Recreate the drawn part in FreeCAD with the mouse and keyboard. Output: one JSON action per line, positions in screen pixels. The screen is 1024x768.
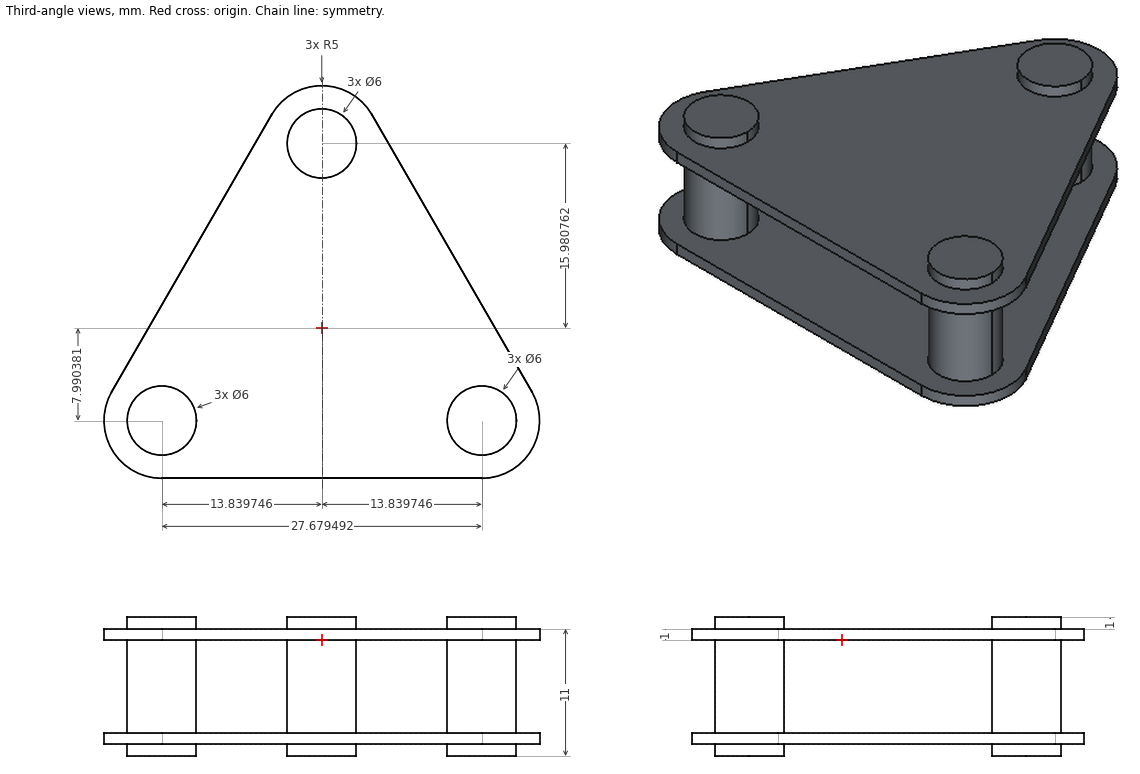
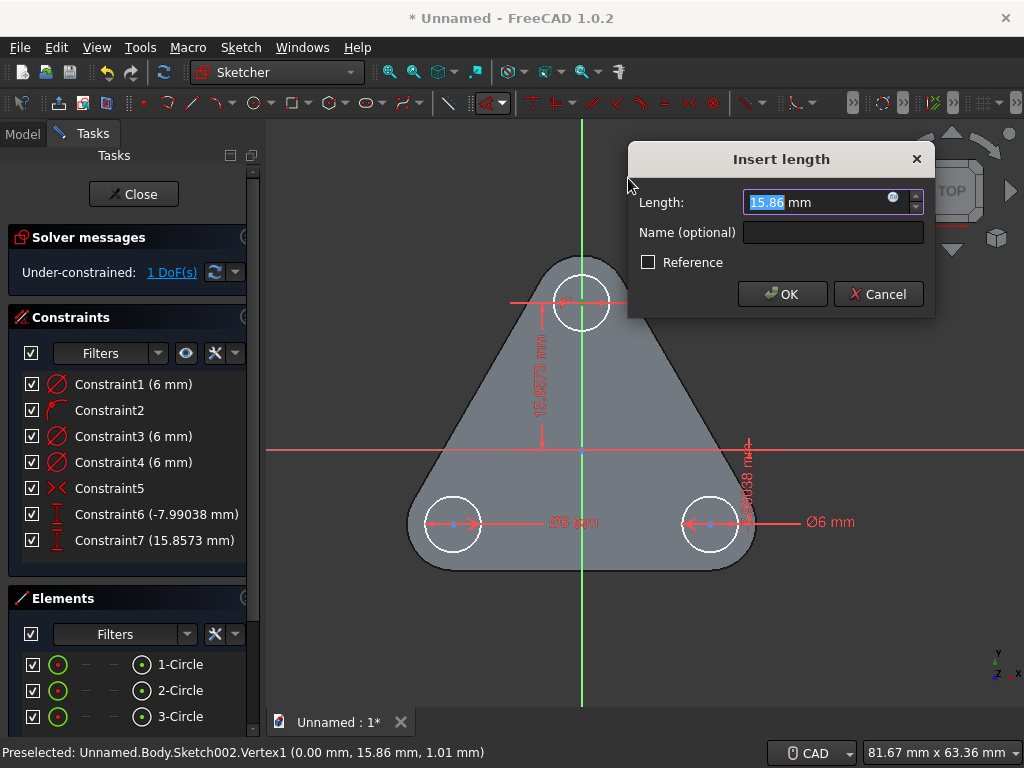
{"action": "type", "text": "15.980762"}
{"action": "key", "text": "Return"}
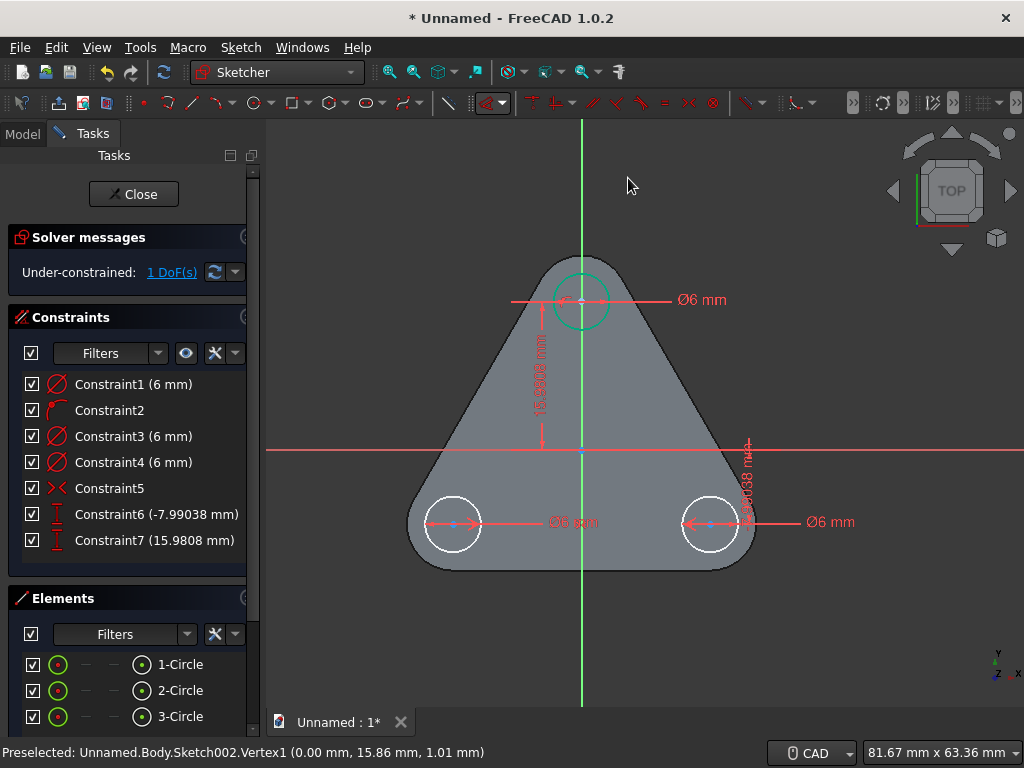
{"action": "left_click", "coordinate": [710, 524]}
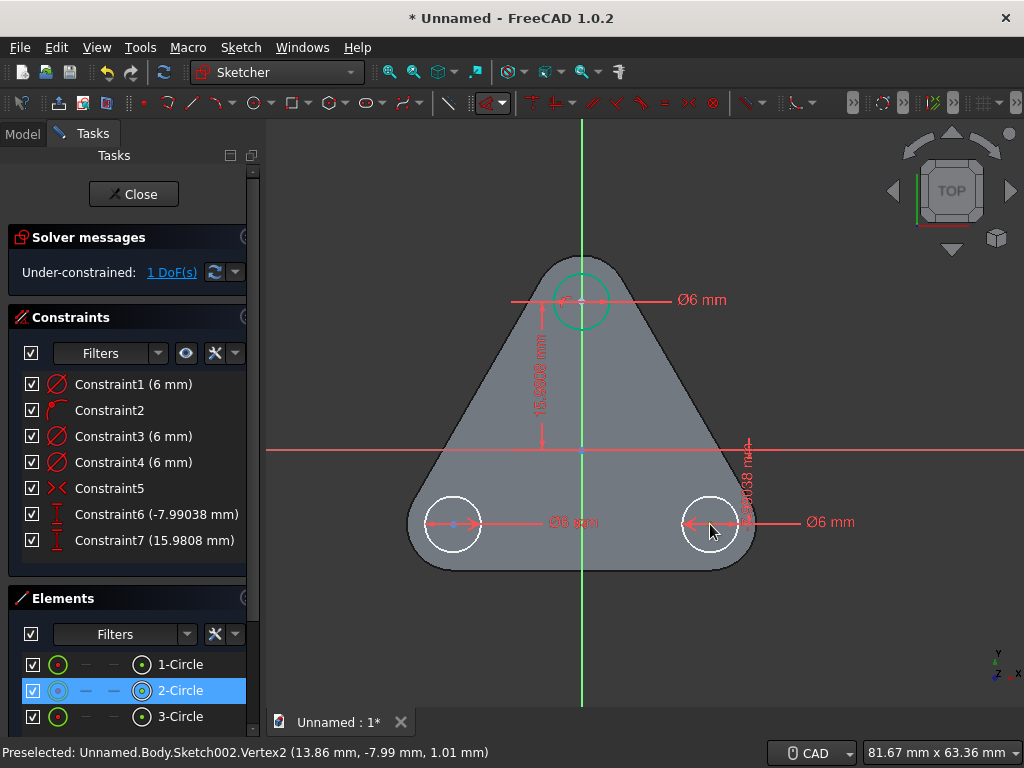
{"action": "left_click", "coordinate": [504, 104]}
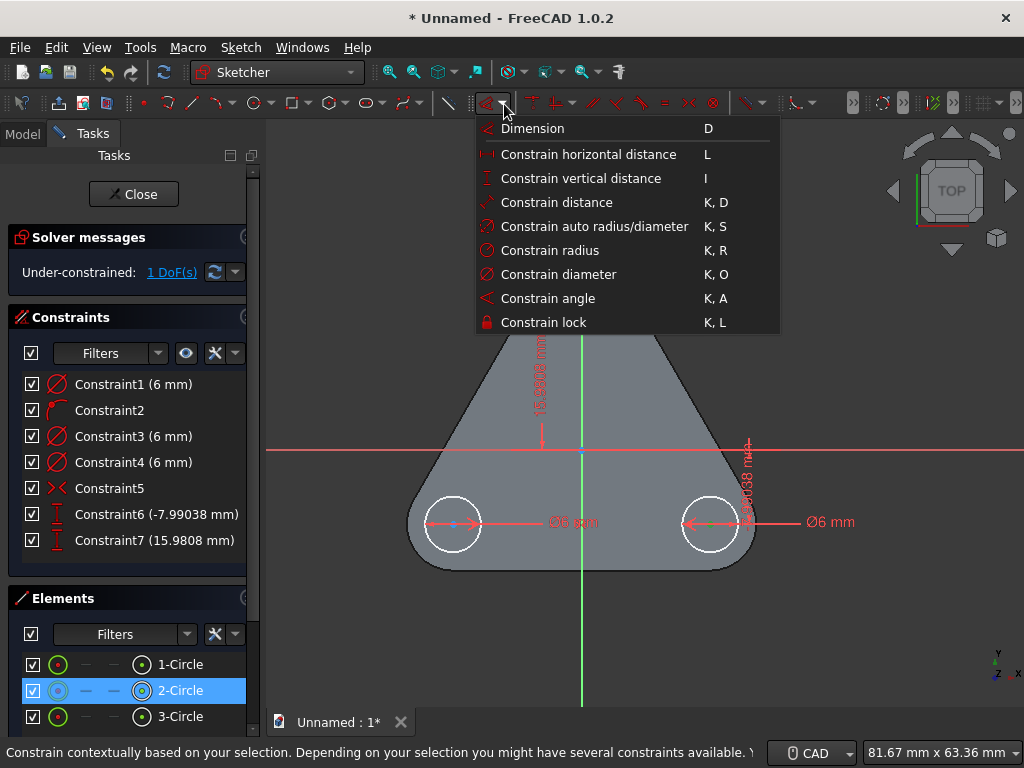
{"action": "left_click", "coordinate": [628, 154]}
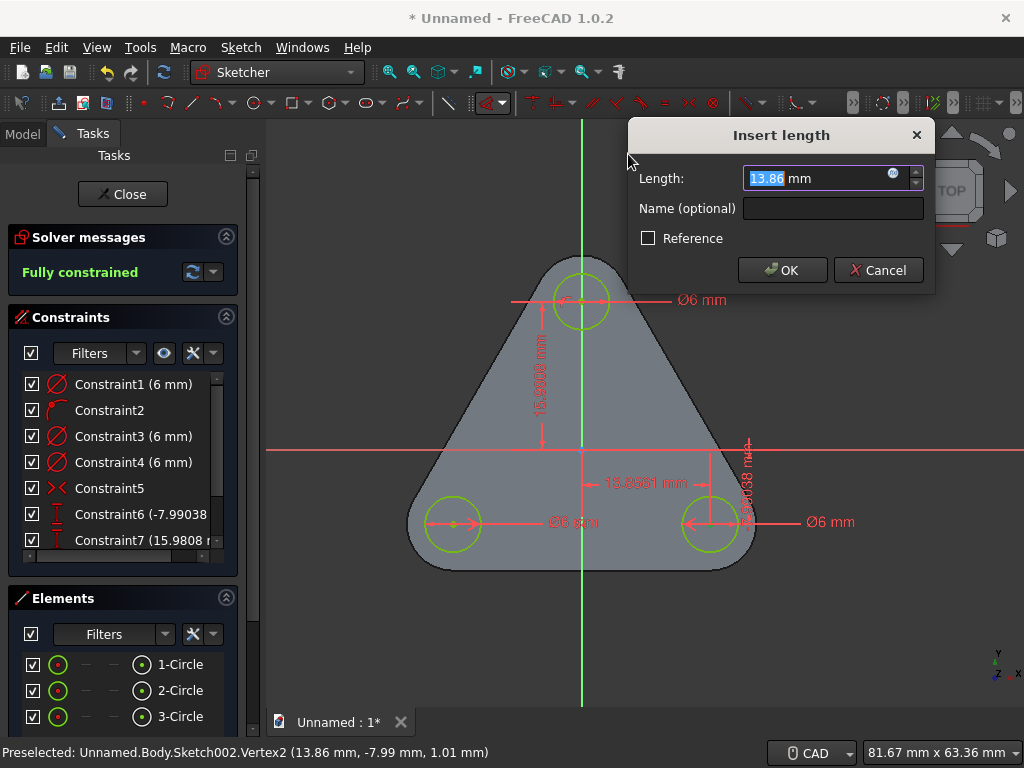
{"action": "type", "text": "13.839746"}
{"action": "key", "text": "Return"}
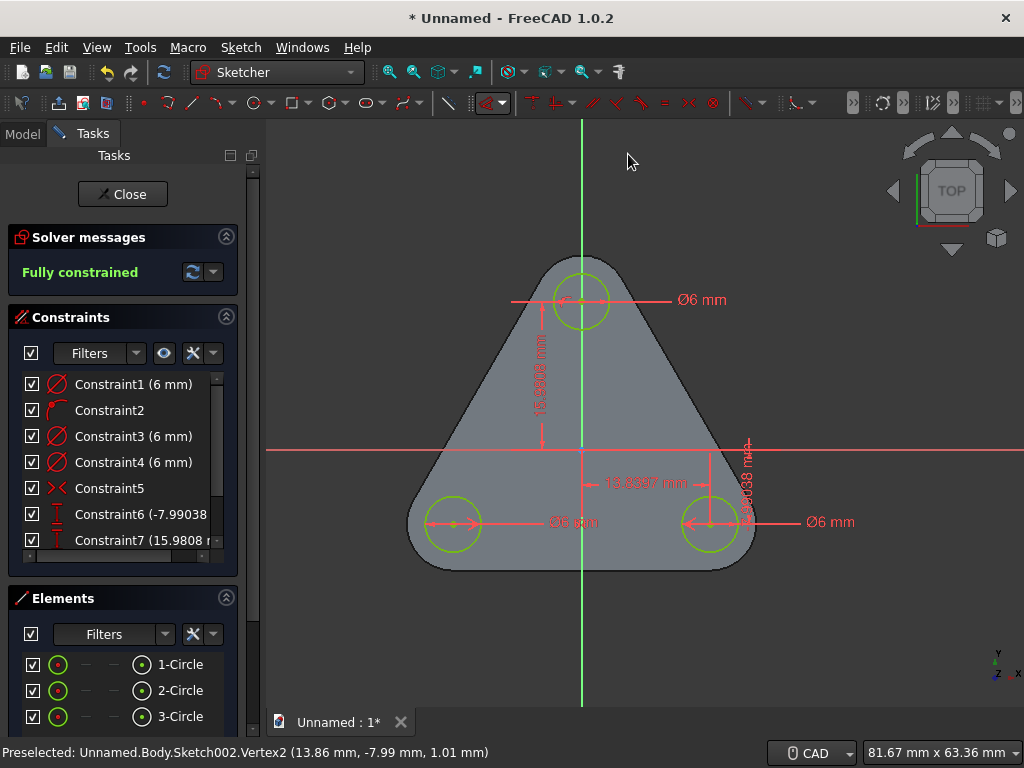
{"action": "left_click", "coordinate": [123, 194]}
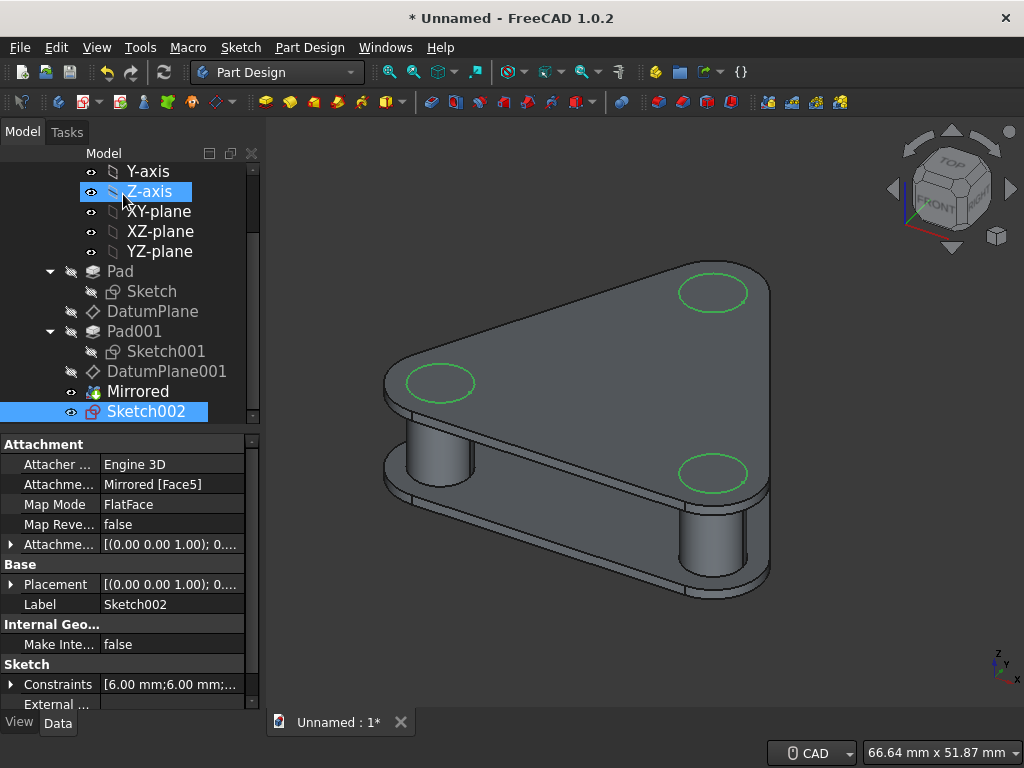
{"action": "left_click", "coordinate": [266, 102]}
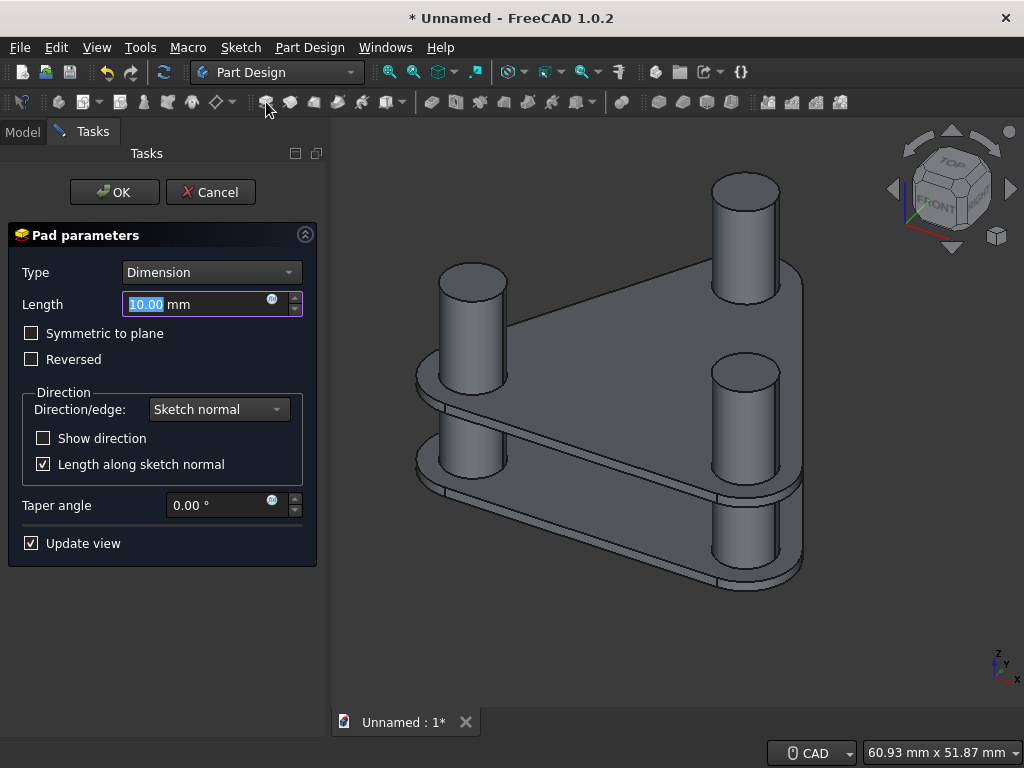
{"action": "type", "text": "1"}
{"action": "key", "text": "Tab"}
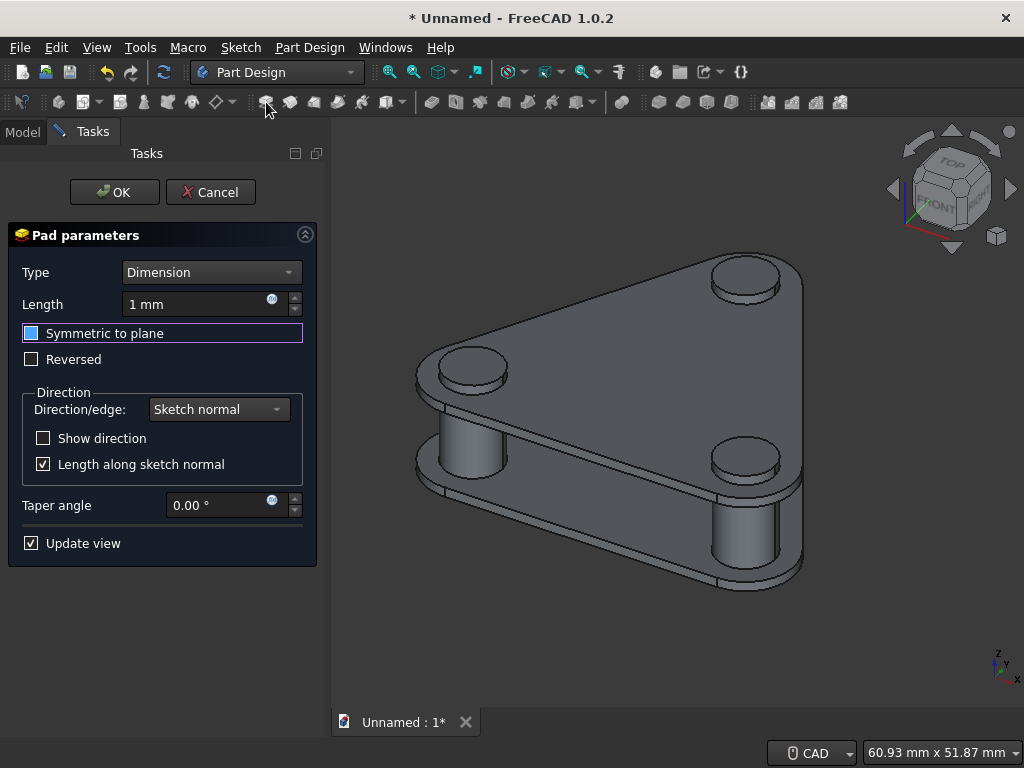
{"action": "left_click", "coordinate": [115, 192]}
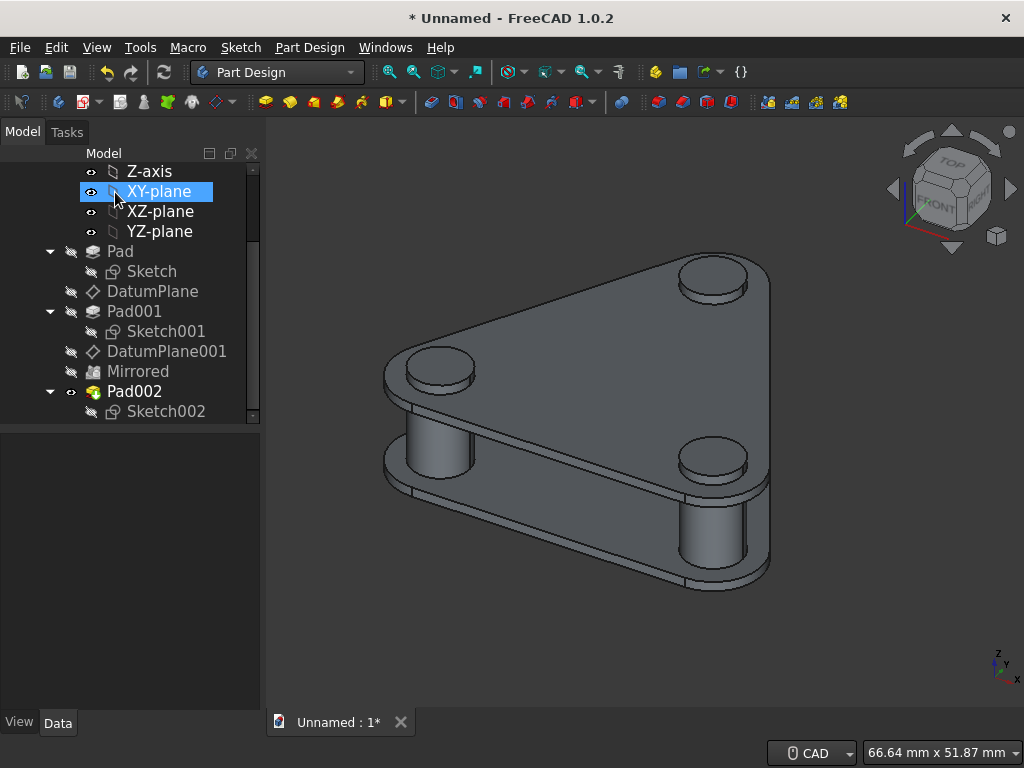
{"action": "key", "text": "0"}